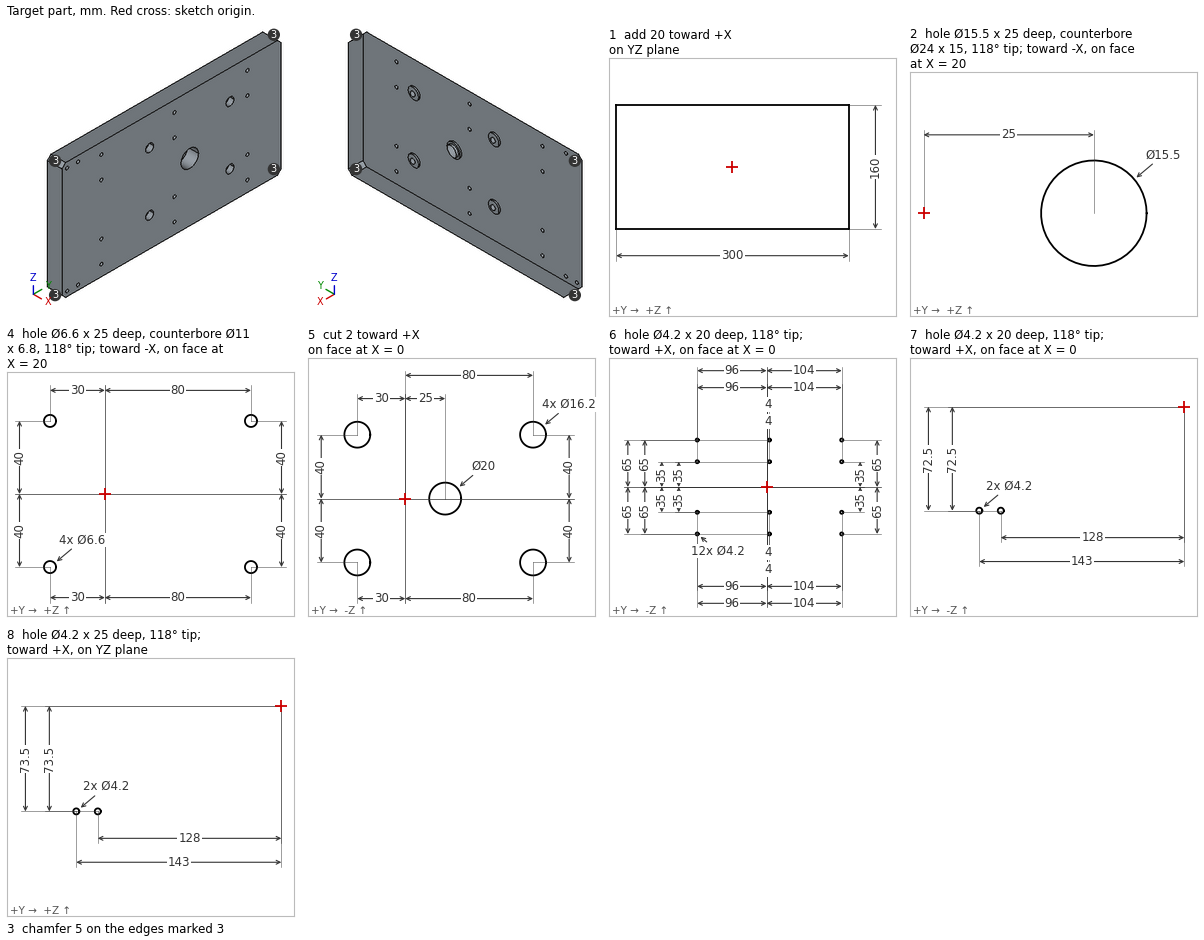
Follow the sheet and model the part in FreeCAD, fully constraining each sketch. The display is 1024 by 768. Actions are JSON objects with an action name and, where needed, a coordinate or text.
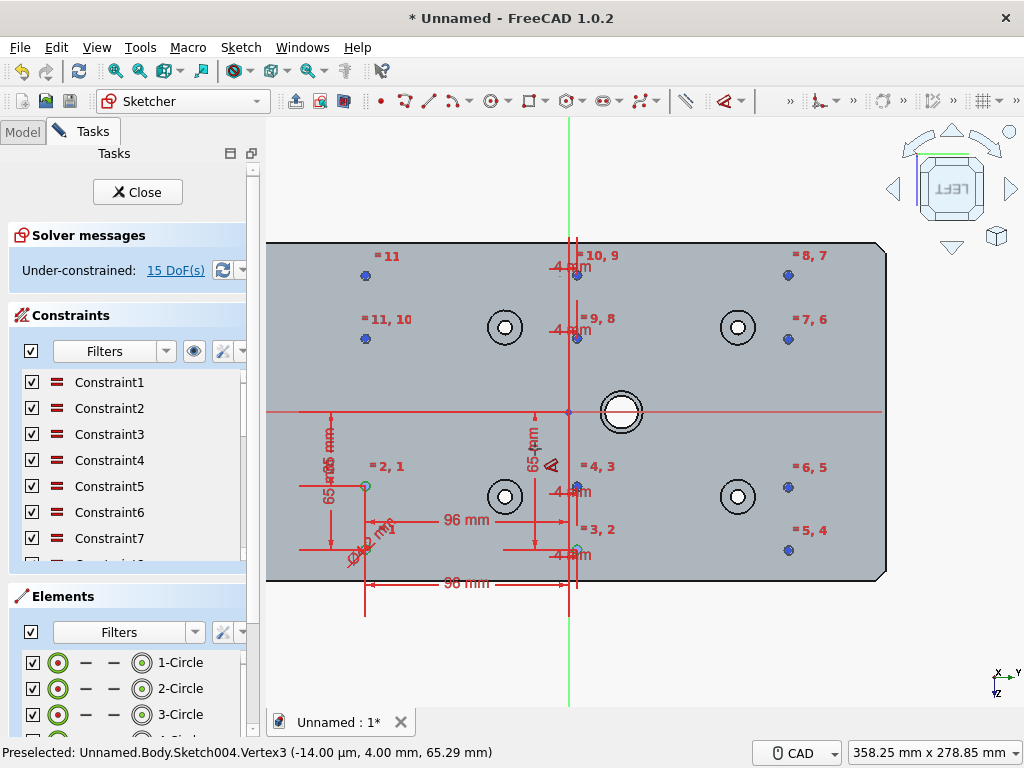
{"action": "left_click", "coordinate": [577, 487]}
{"action": "left_click", "coordinate": [611, 450]}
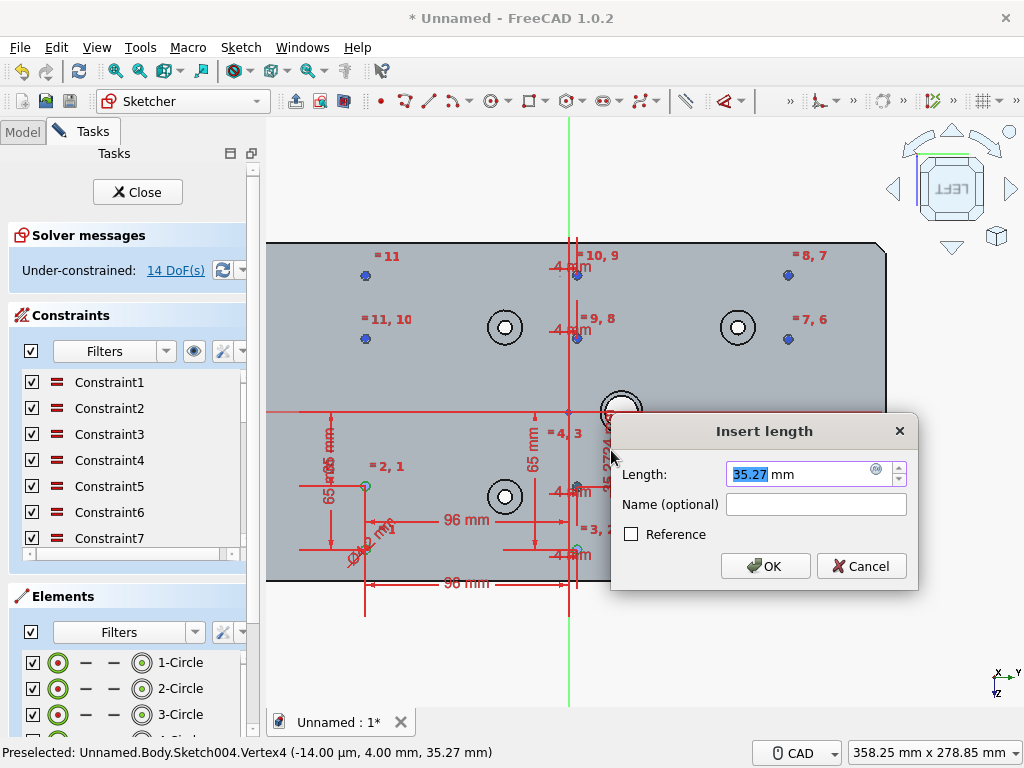
{"action": "type", "text": "35"}
{"action": "key", "text": "Return"}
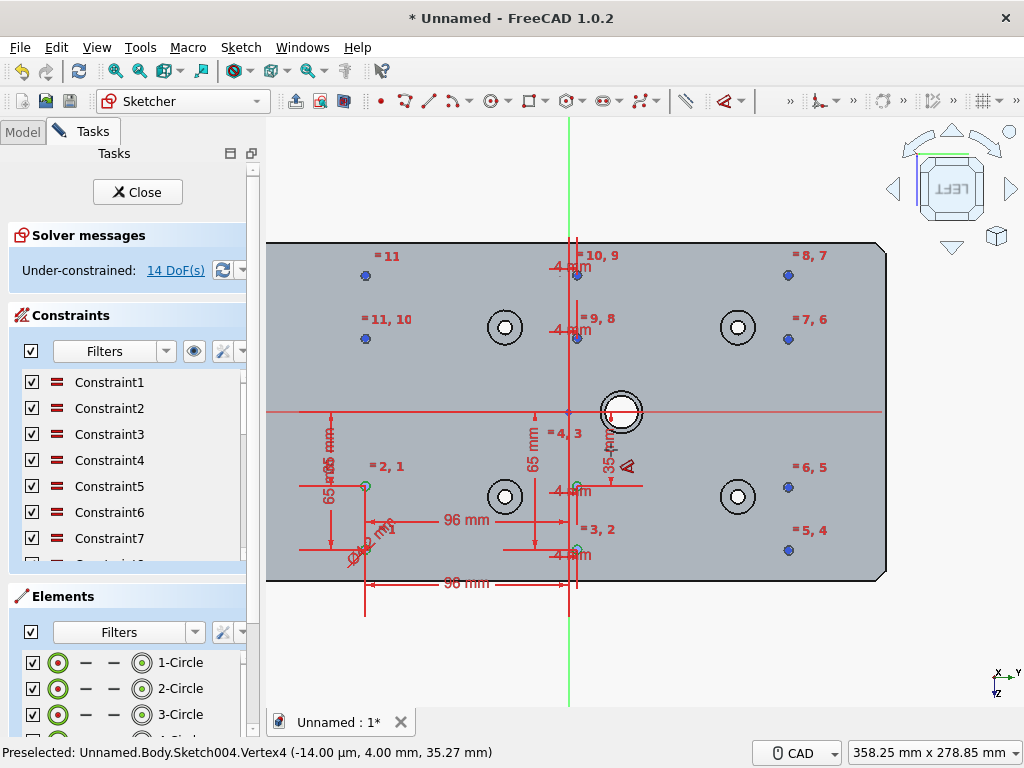
{"action": "left_click", "coordinate": [789, 550]}
{"action": "left_click", "coordinate": [823, 481]}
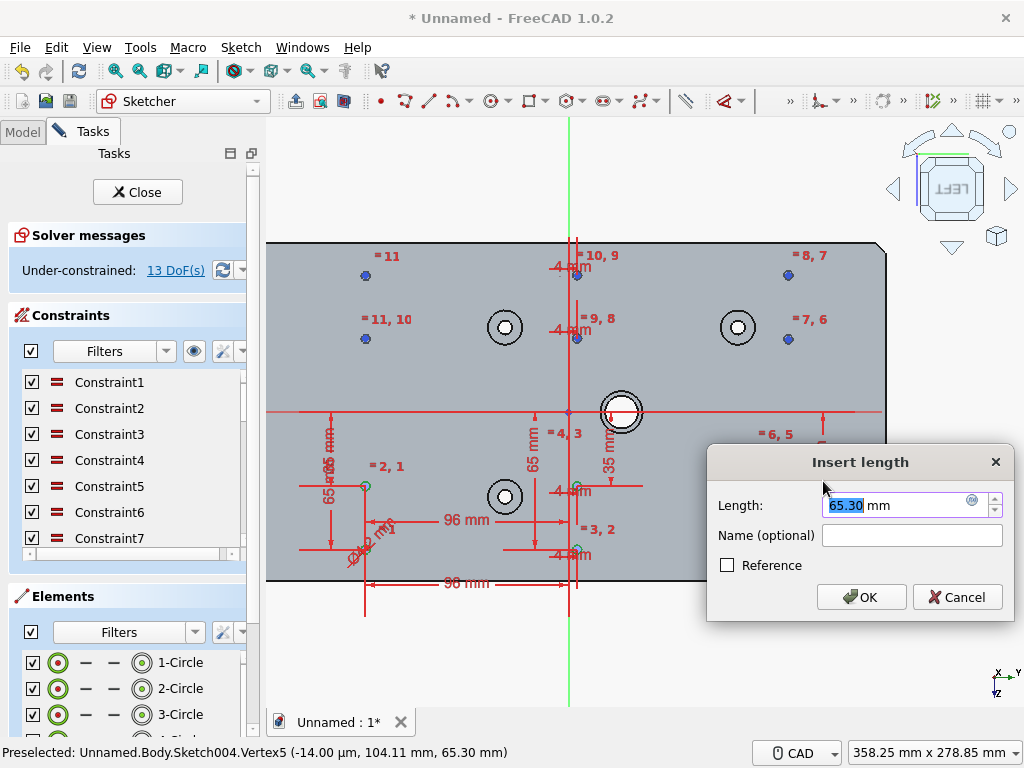
{"action": "type", "text": "65"}
{"action": "key", "text": "Return"}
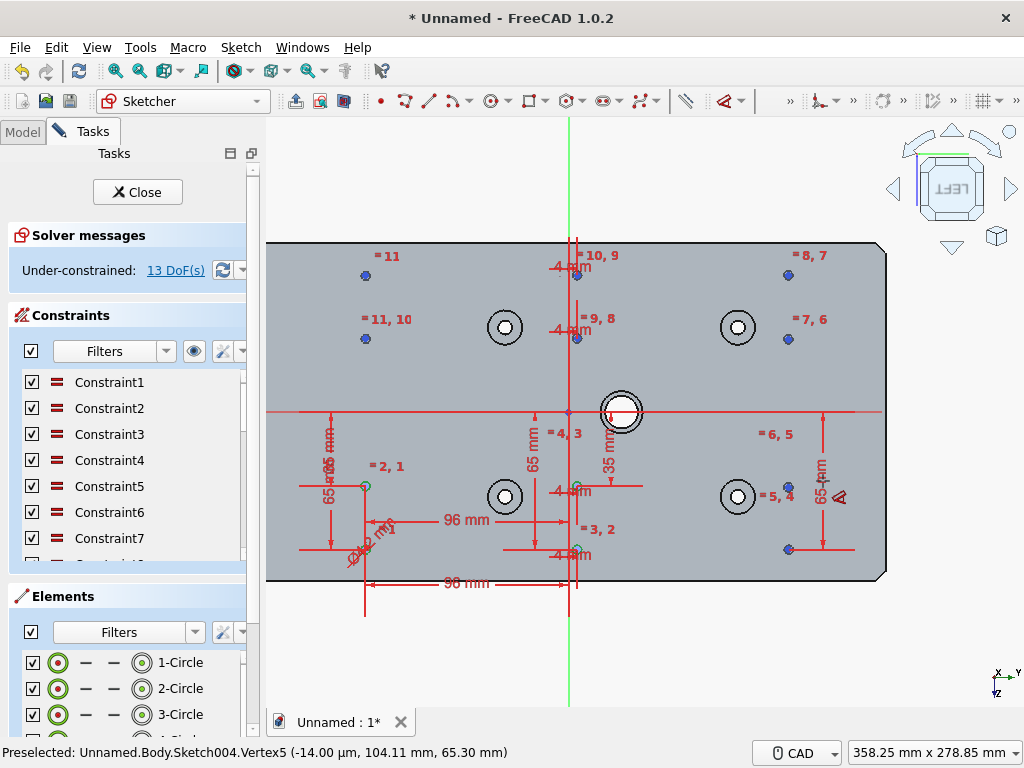
{"action": "left_click", "coordinate": [788, 487]}
{"action": "left_click", "coordinate": [822, 450]}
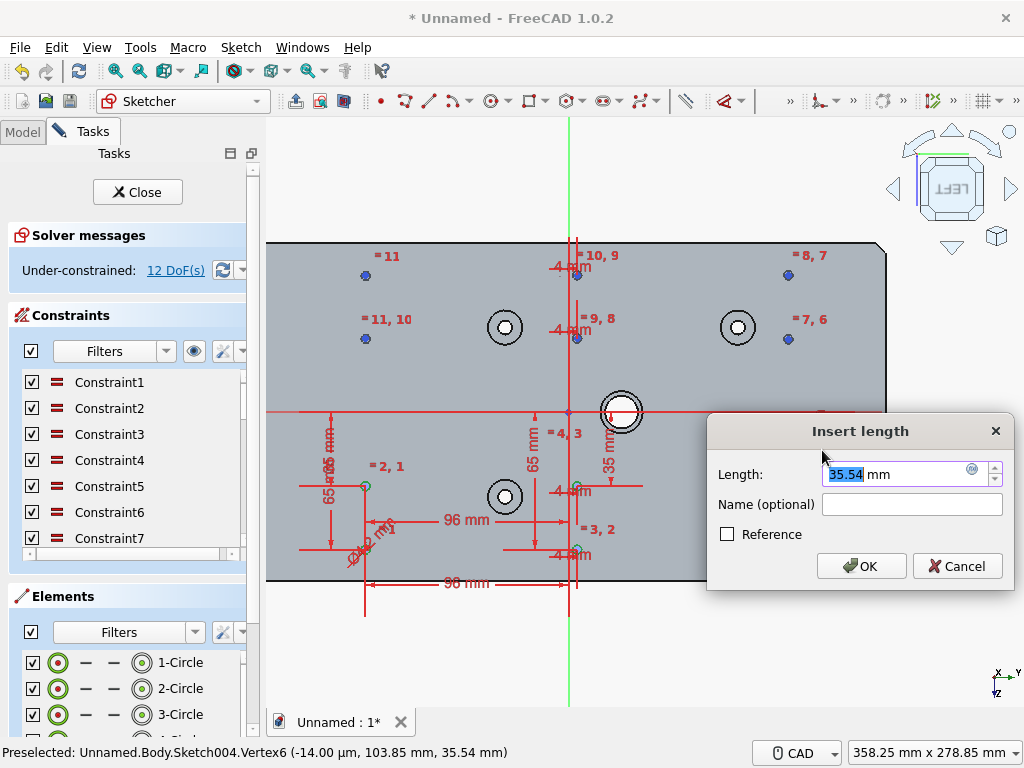
{"action": "type", "text": "35"}
{"action": "key", "text": "Return"}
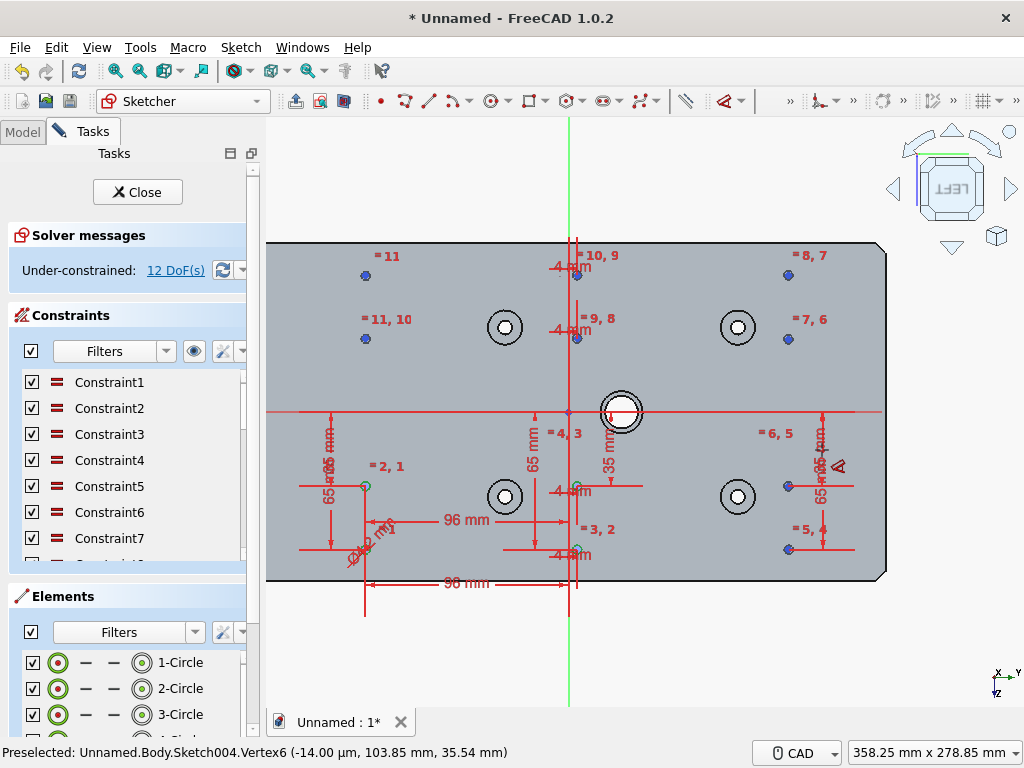
{"action": "left_click", "coordinate": [788, 339]}
{"action": "left_click", "coordinate": [822, 376]}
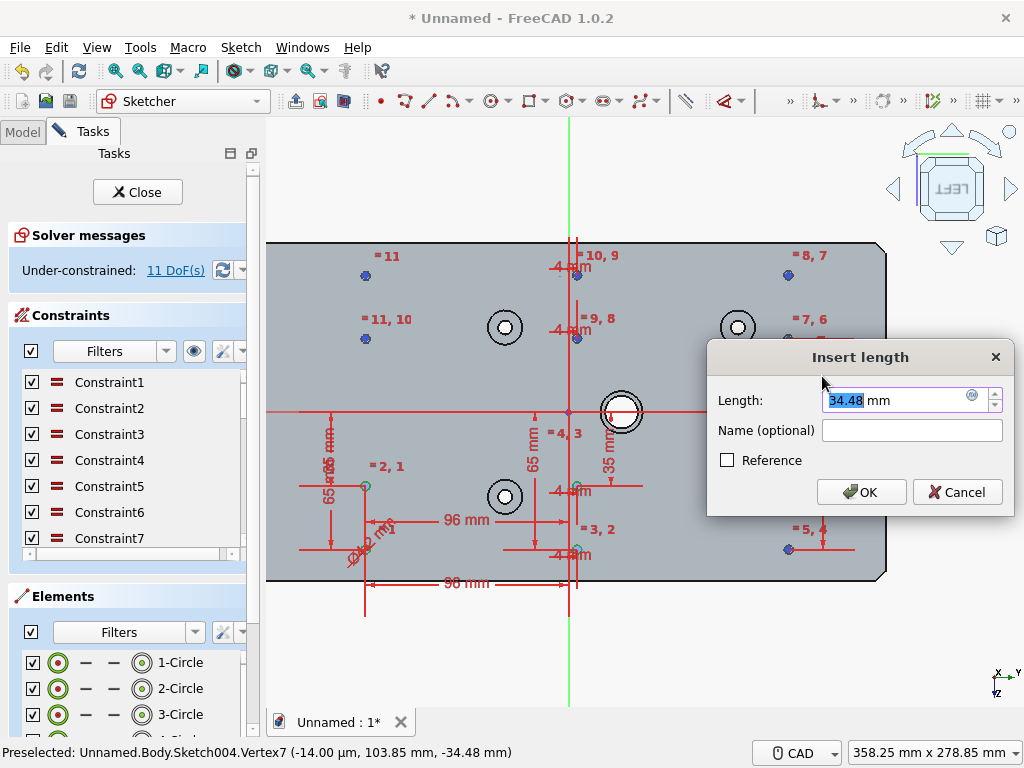
{"action": "type", "text": "35"}
{"action": "key", "text": "Return"}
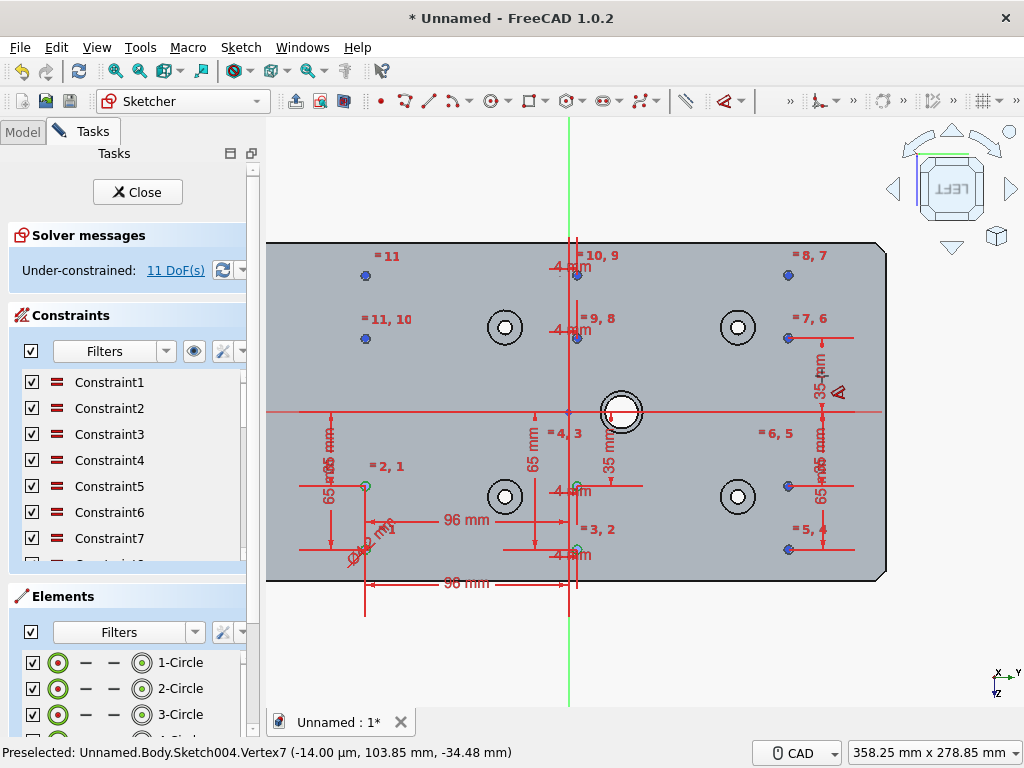
{"action": "left_click", "coordinate": [788, 275]}
{"action": "left_click", "coordinate": [822, 344]}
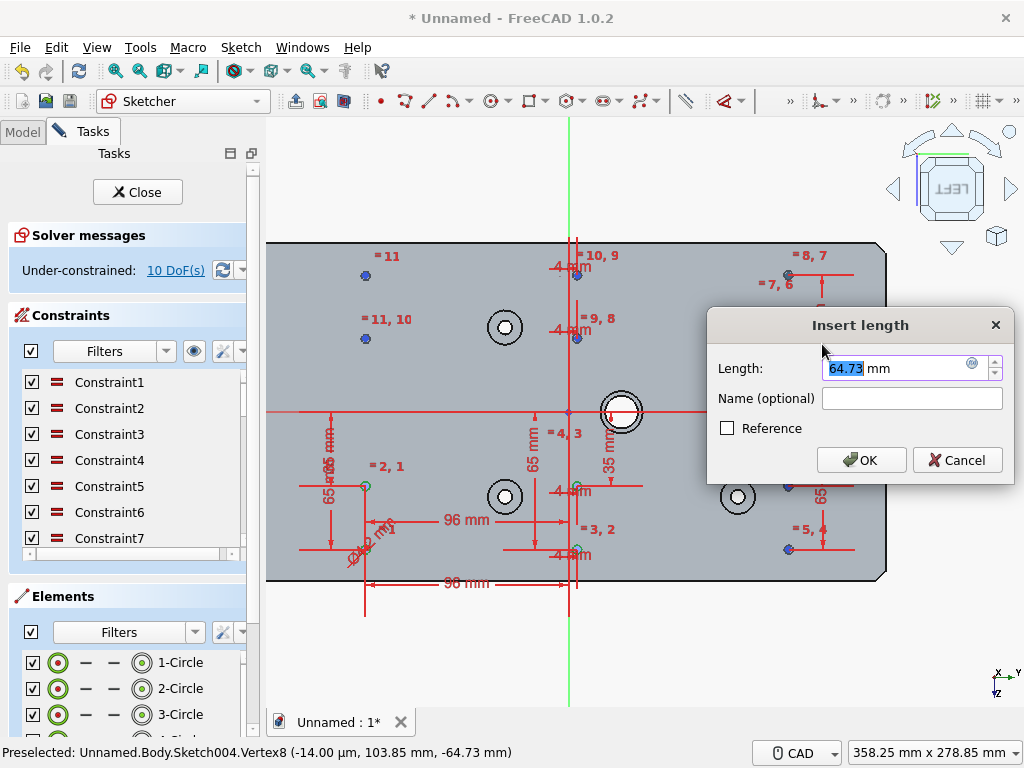
{"action": "type", "text": "65"}
{"action": "key", "text": "Return"}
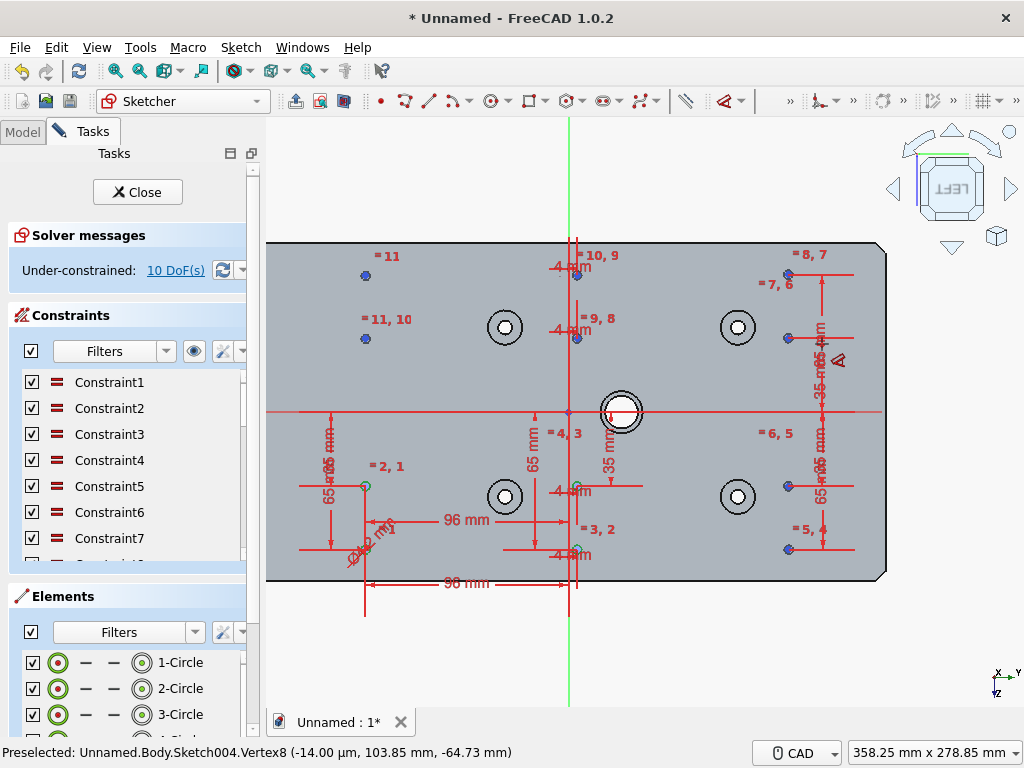
{"action": "left_click", "coordinate": [577, 338]}
{"action": "left_click", "coordinate": [535, 375]}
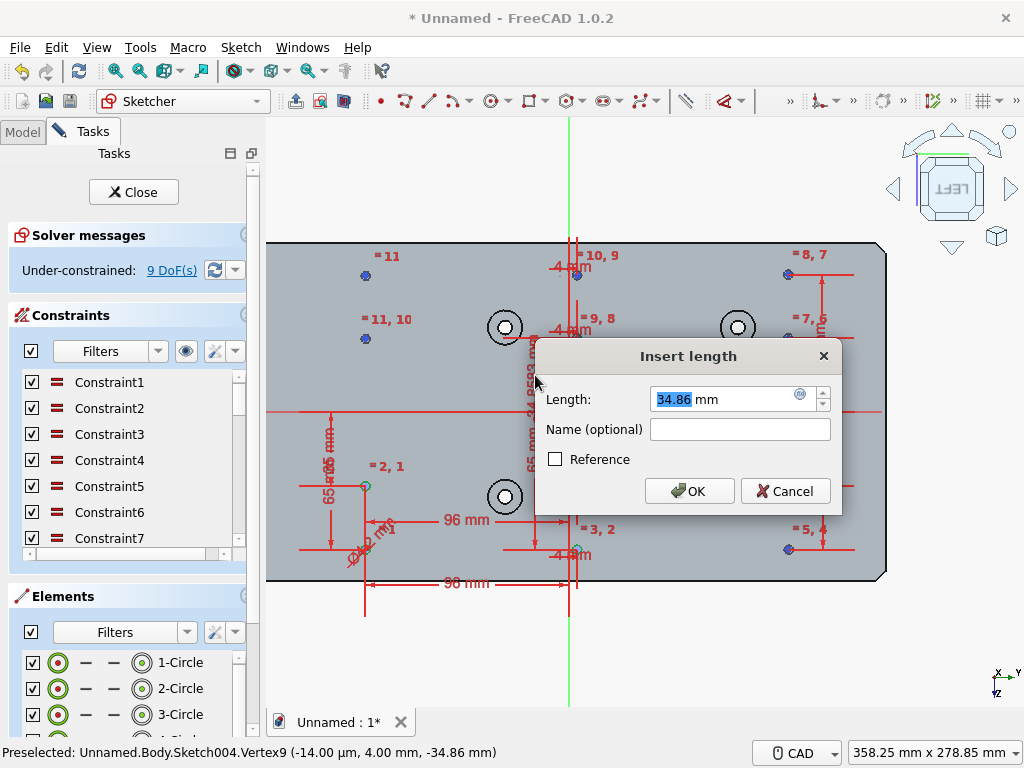
{"action": "type", "text": "35"}
{"action": "key", "text": "Return"}